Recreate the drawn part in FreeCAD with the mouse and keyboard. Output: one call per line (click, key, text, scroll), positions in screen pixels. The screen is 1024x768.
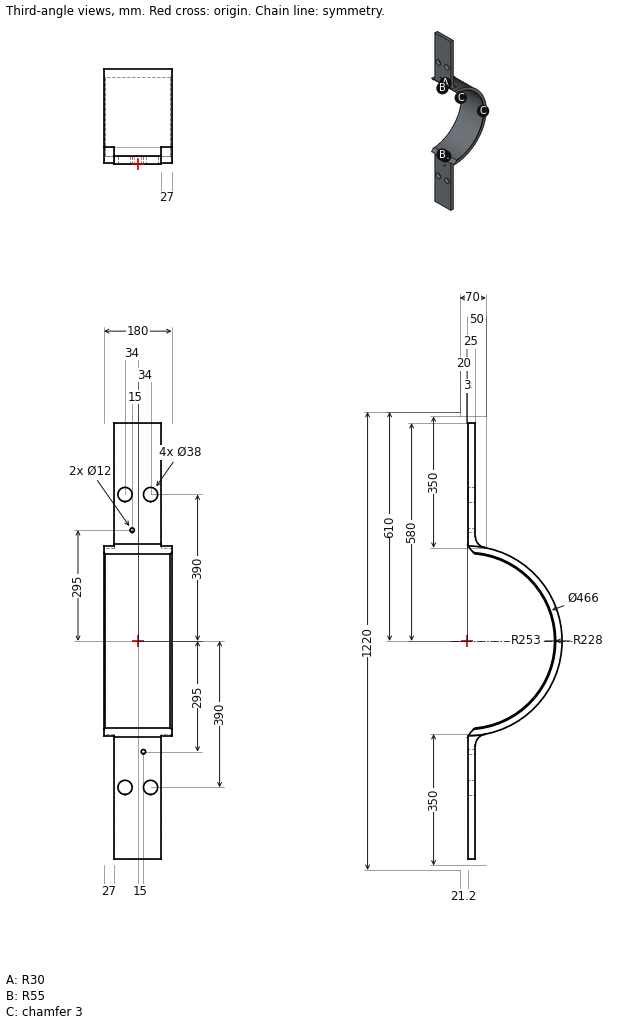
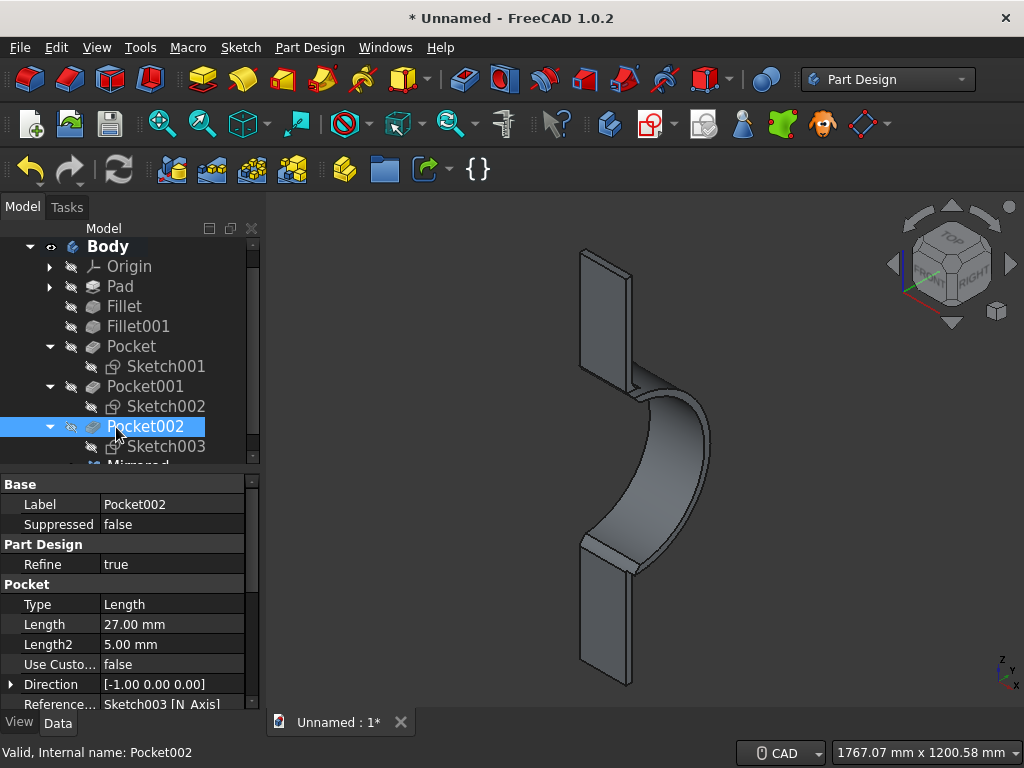
click(172, 170)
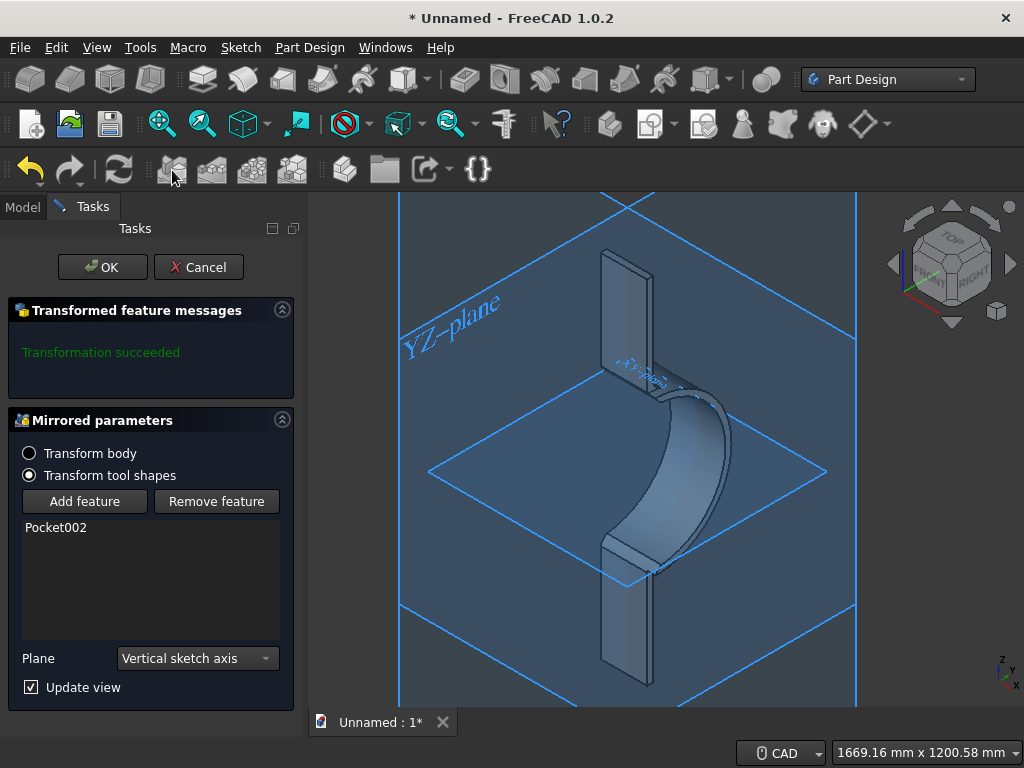
click(198, 658)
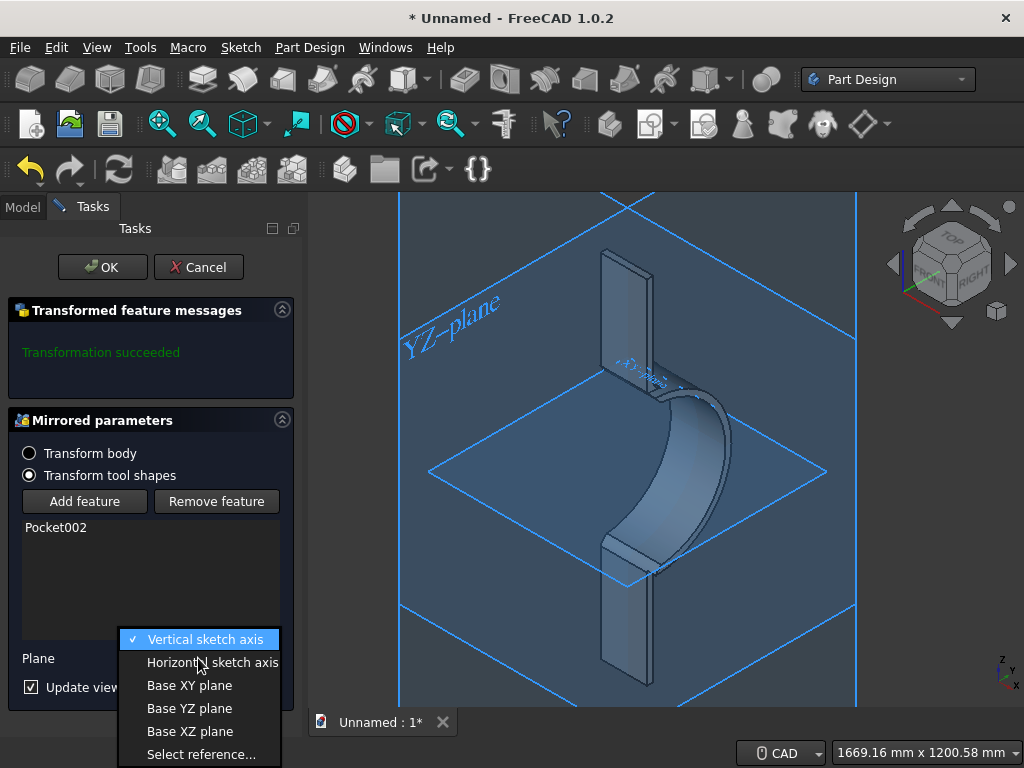
click(198, 708)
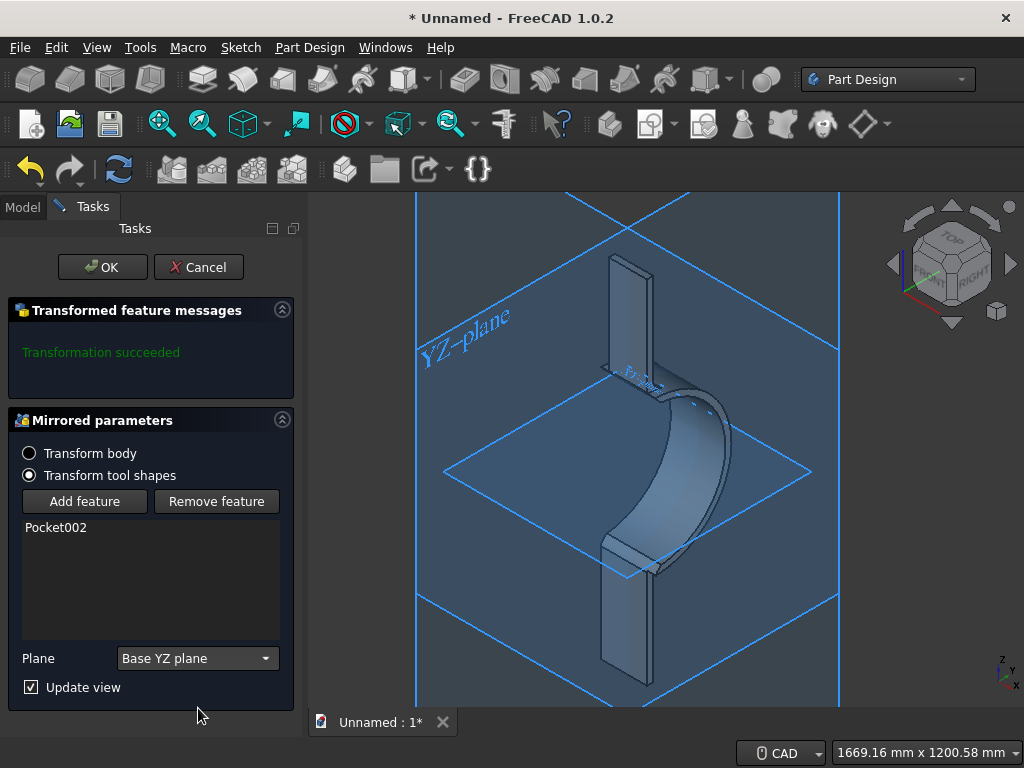
click(103, 267)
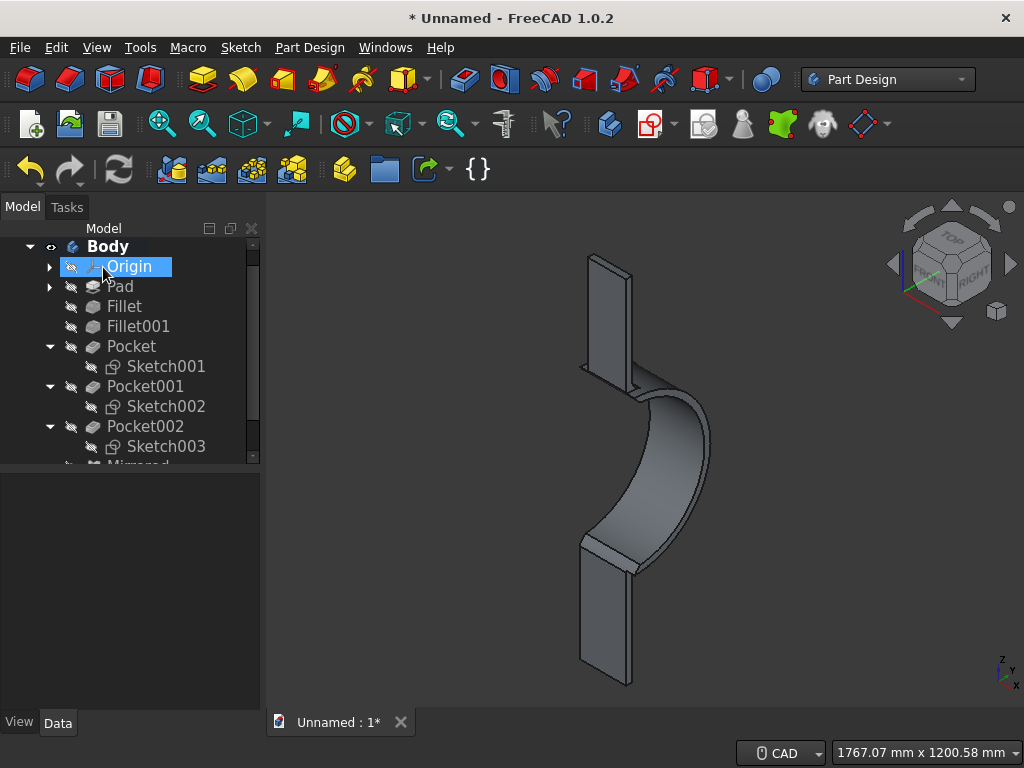
key(6)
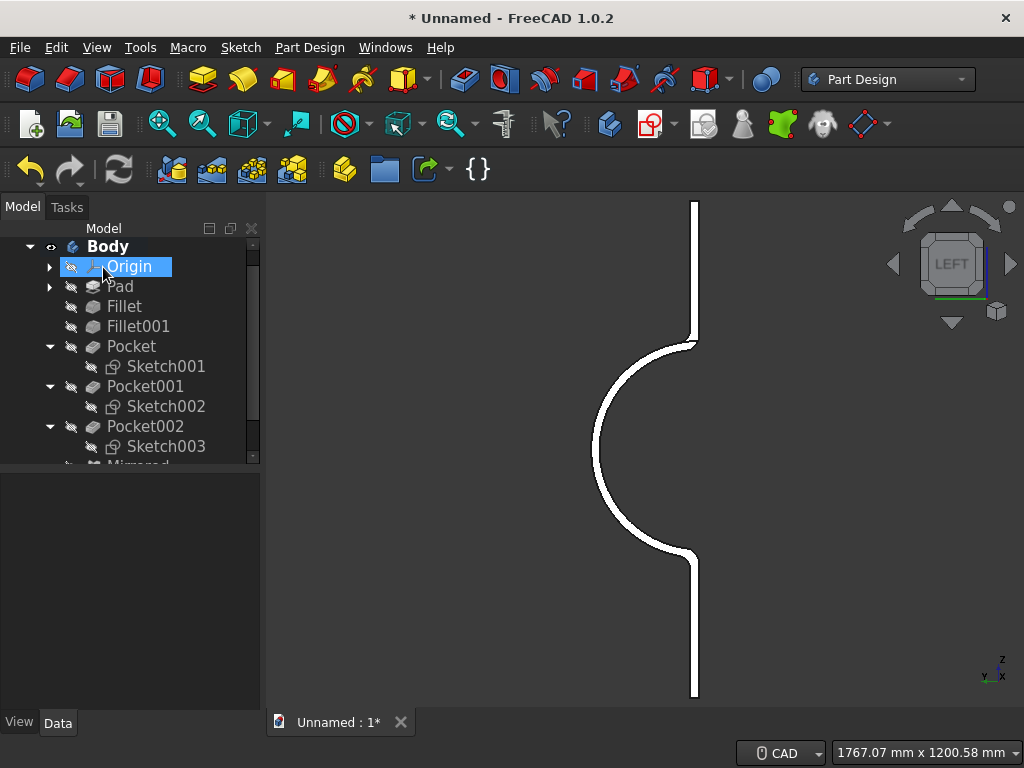
scroll(599, 417, up, 8)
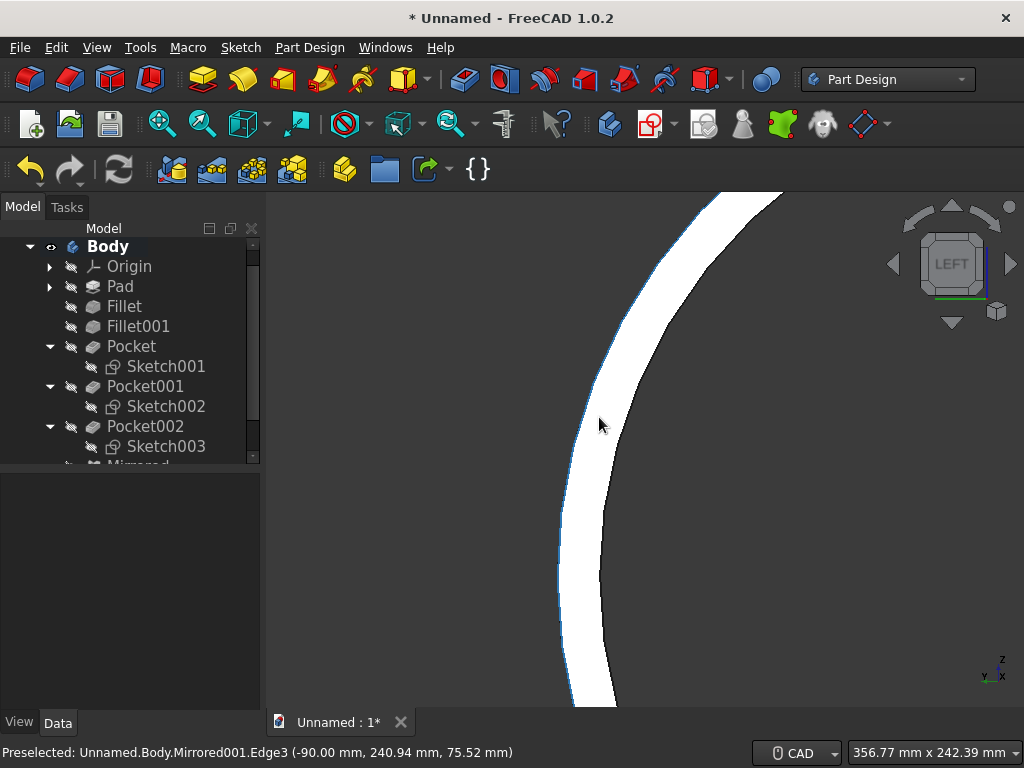
click(596, 417)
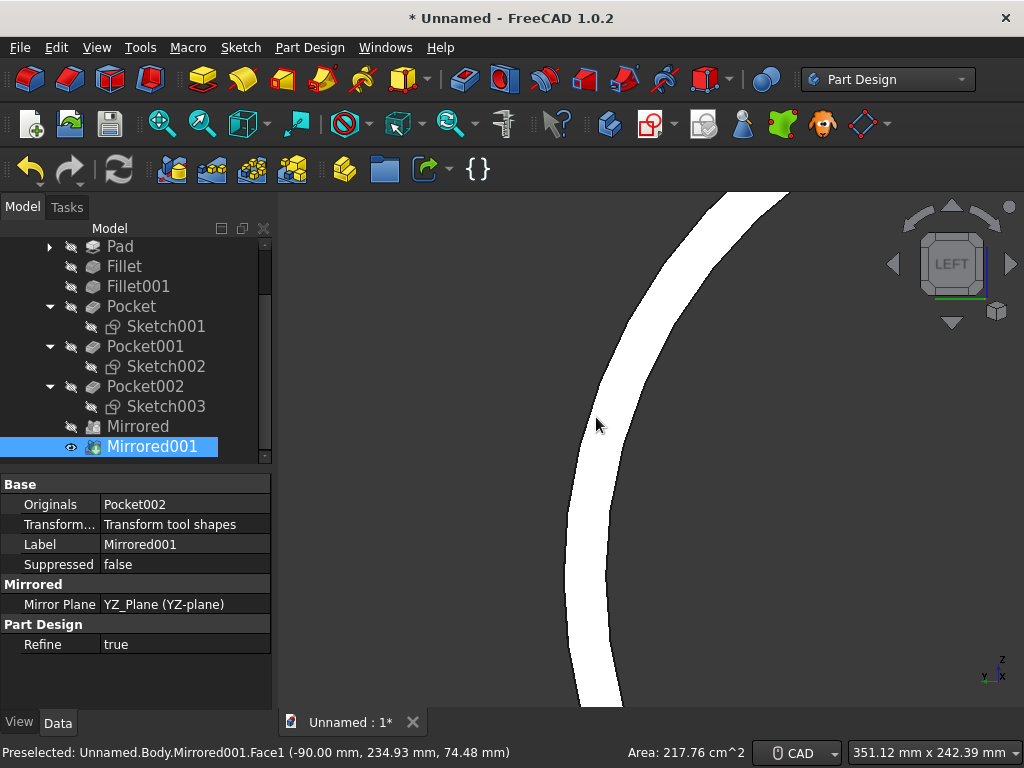
click(650, 124)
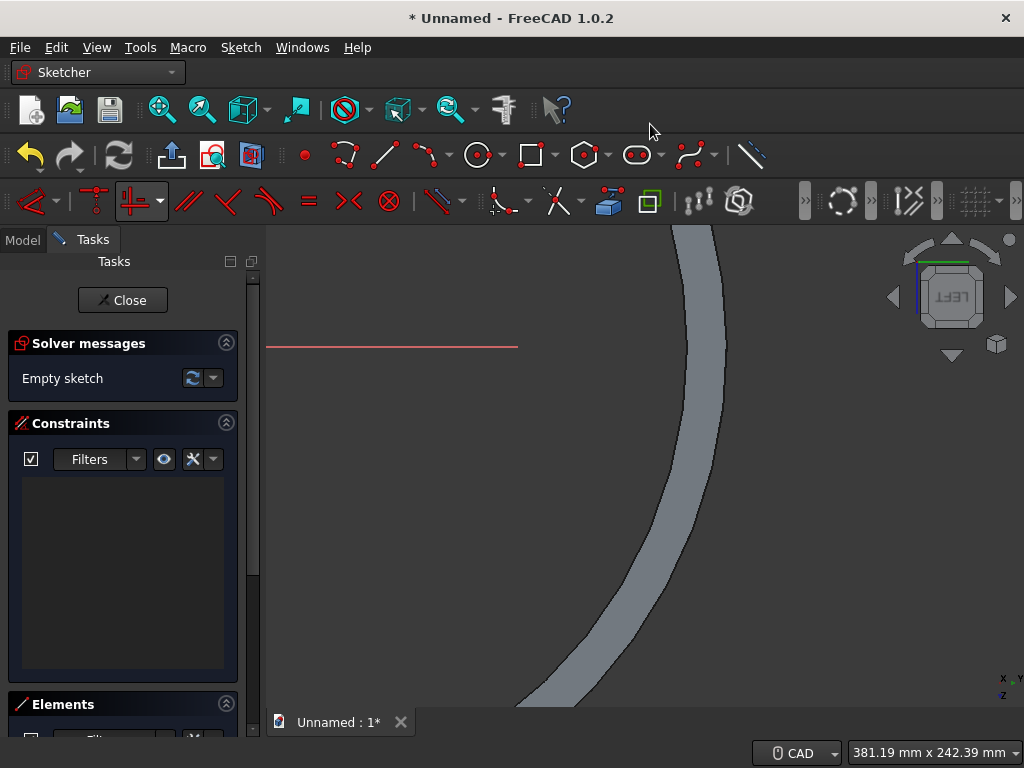
scroll(682, 679, down, 7)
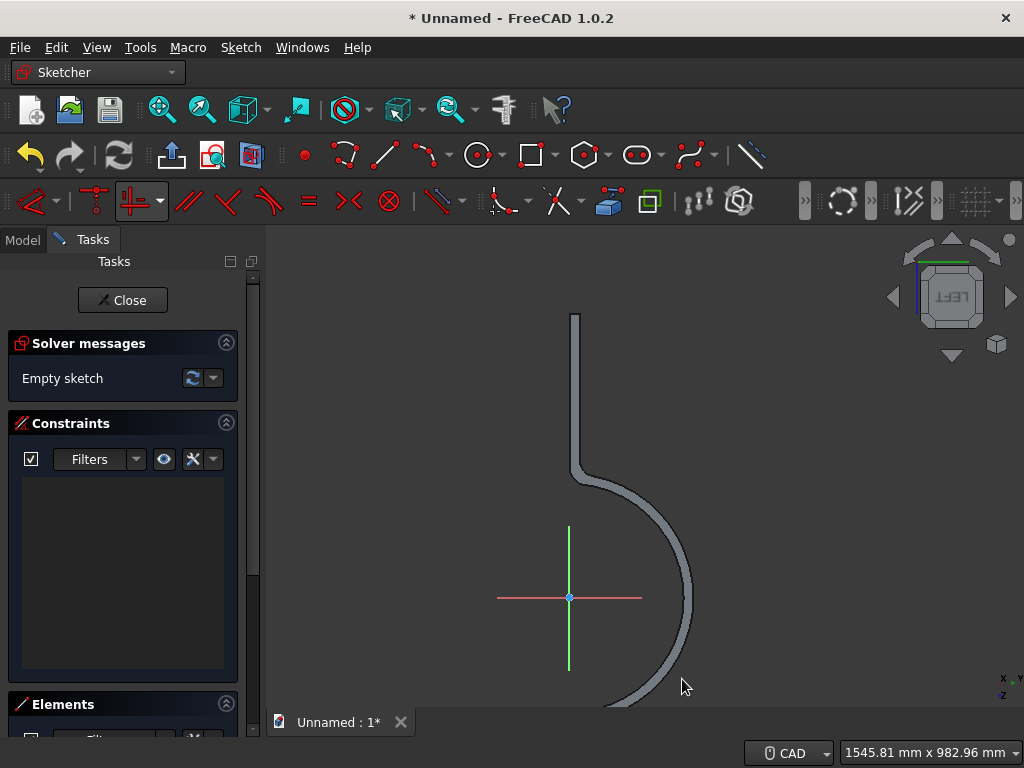
click(346, 156)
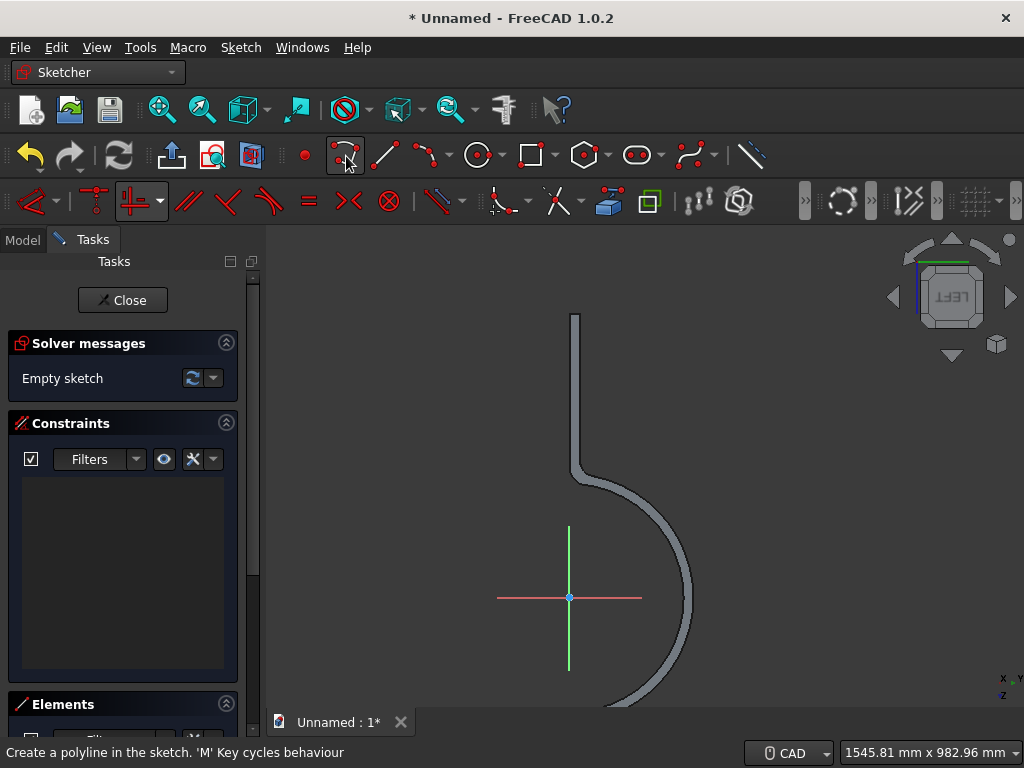
click(594, 476)
click(594, 305)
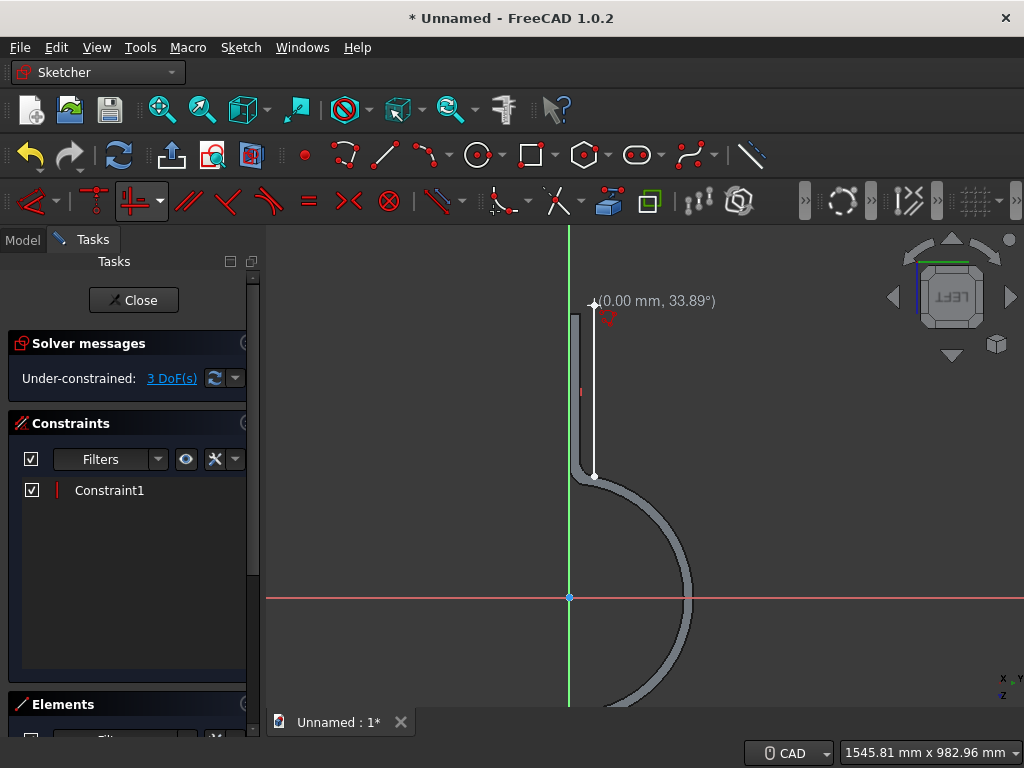
scroll(560, 305, up, 3)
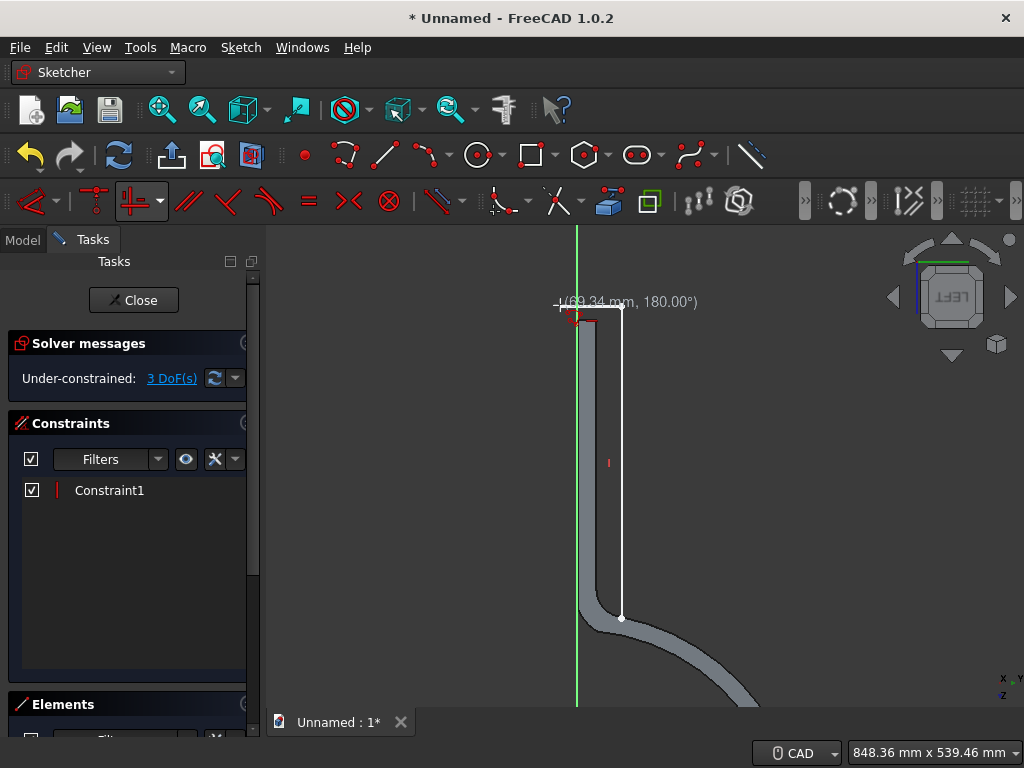
click(559, 305)
click(559, 613)
right_click(559, 613)